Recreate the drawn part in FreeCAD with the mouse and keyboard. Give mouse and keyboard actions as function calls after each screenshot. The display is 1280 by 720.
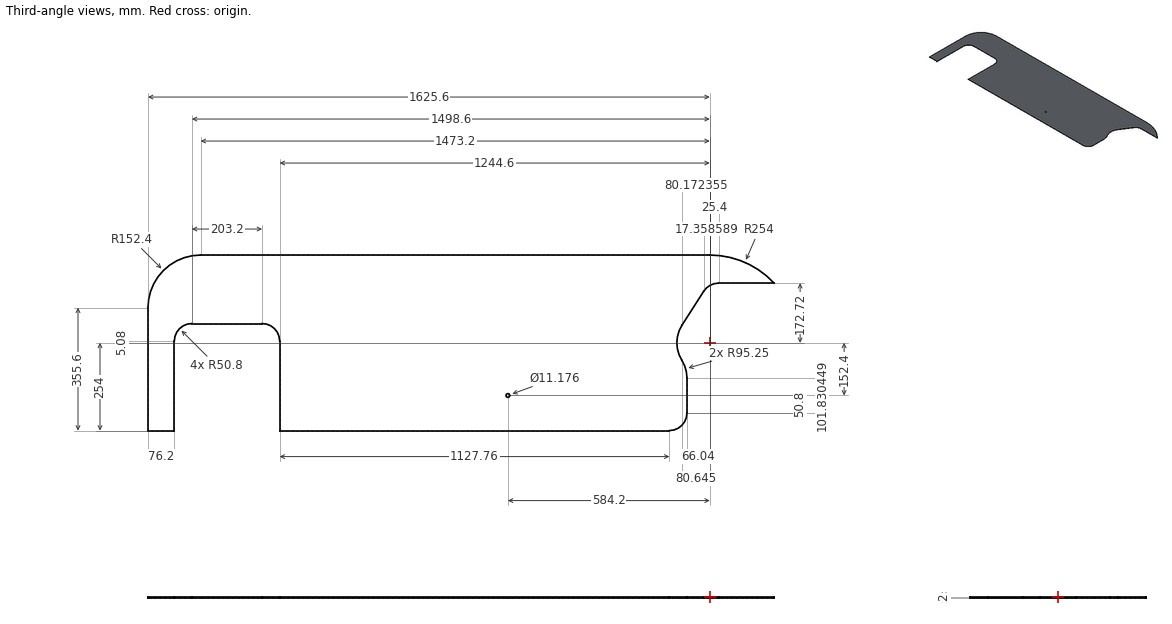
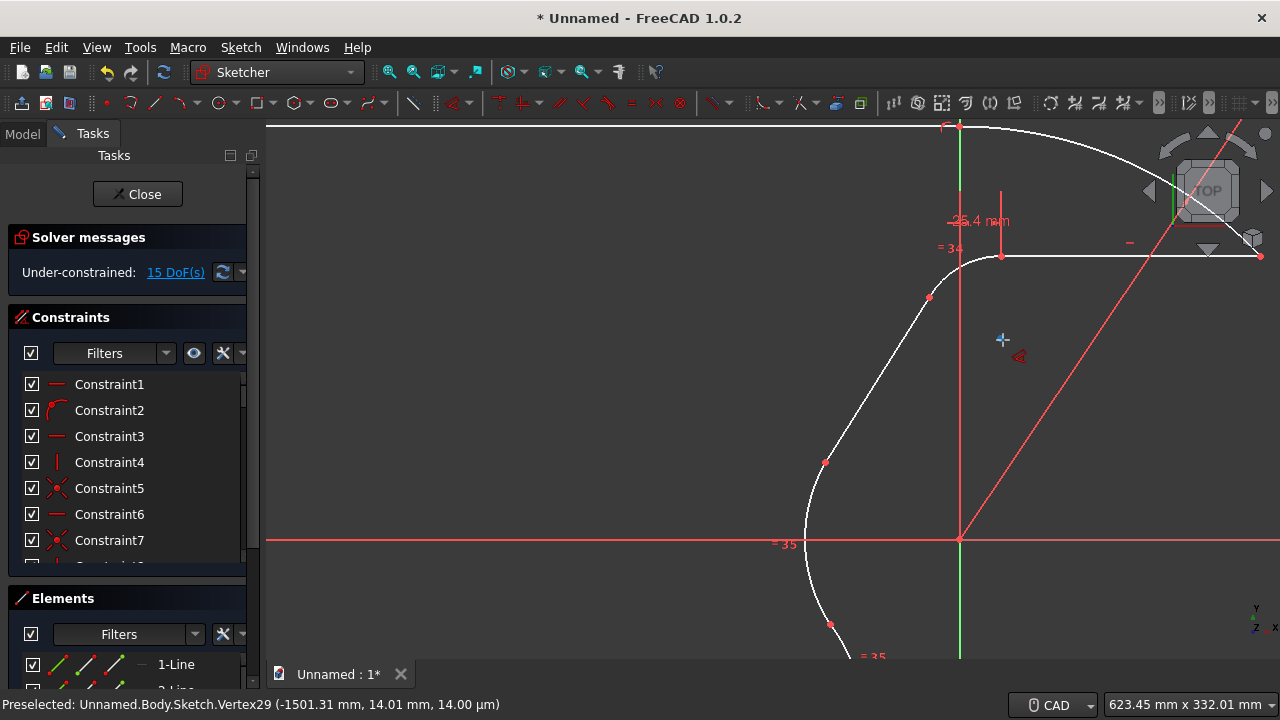
click(1001, 339)
click(980, 305)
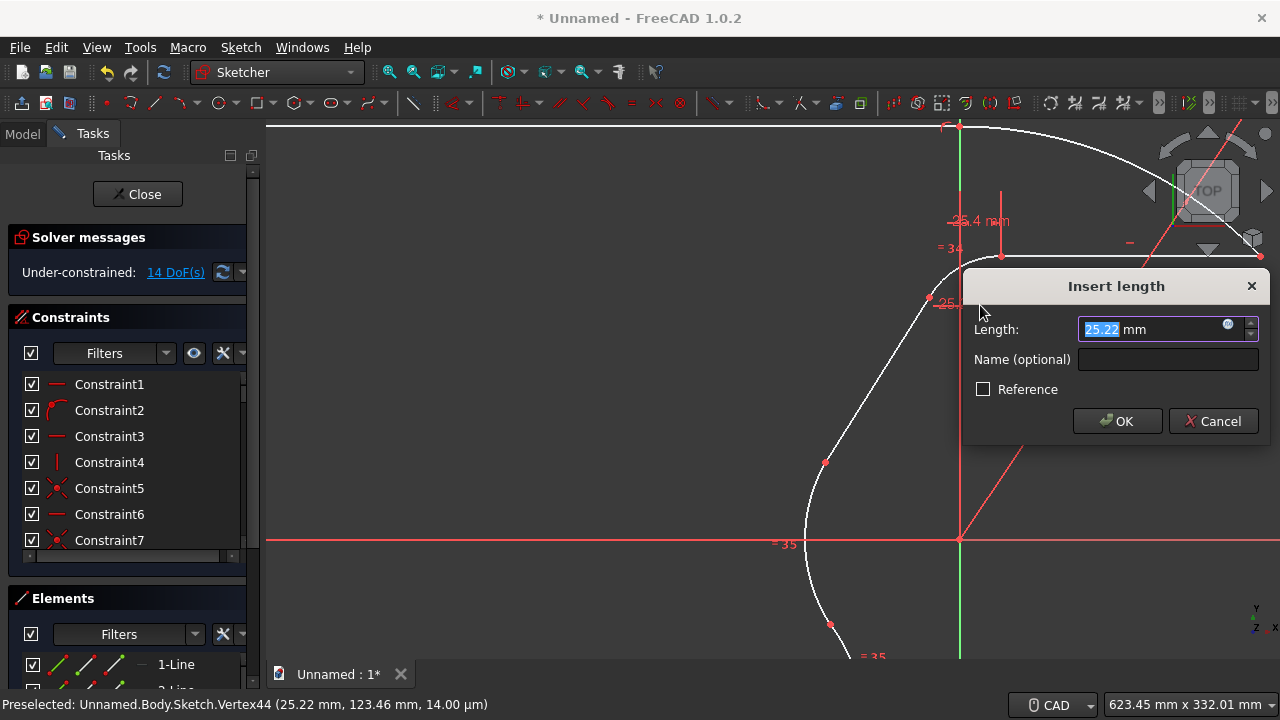
text(25.4)
key(Return)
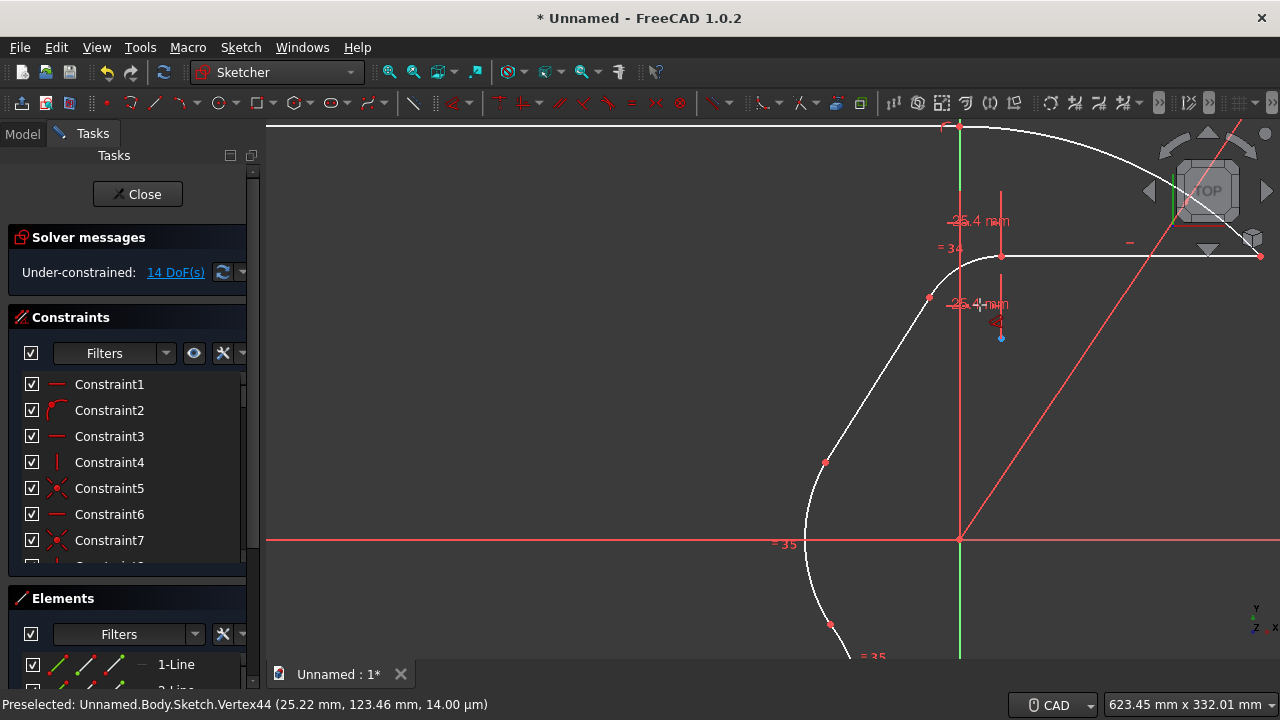
scroll(936, 351, down, 8)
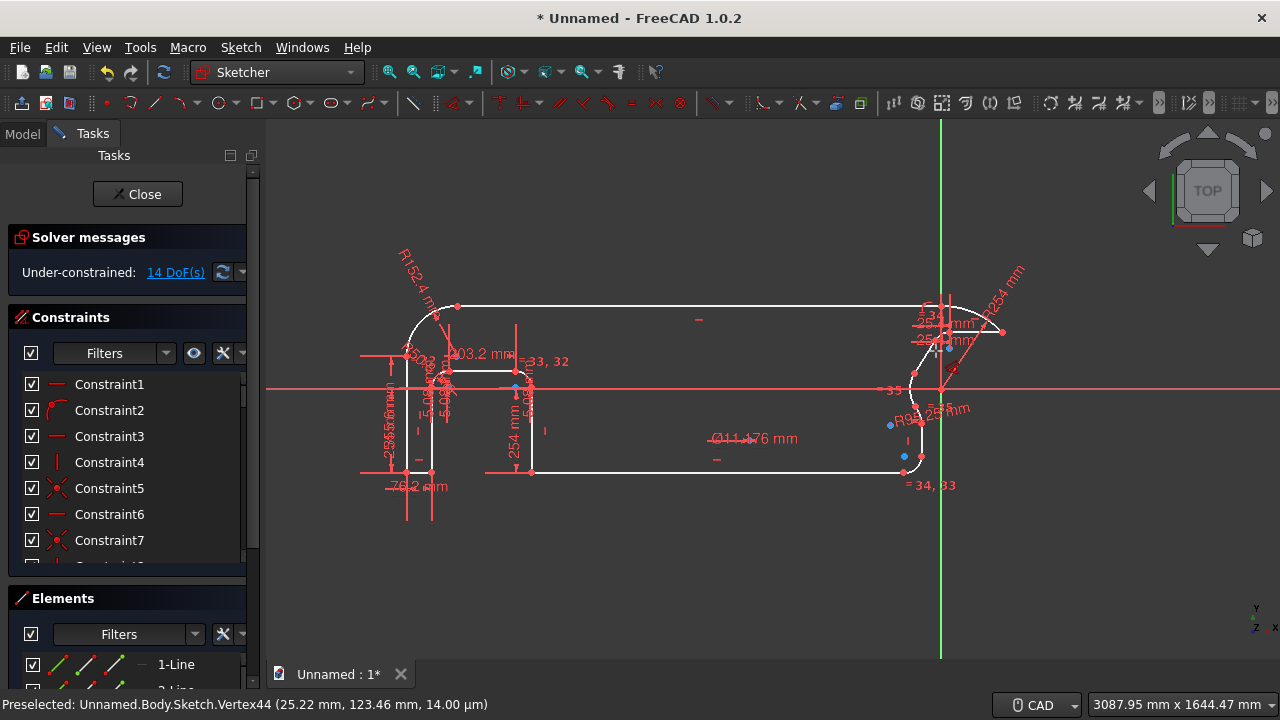
click(750, 441)
click(846, 355)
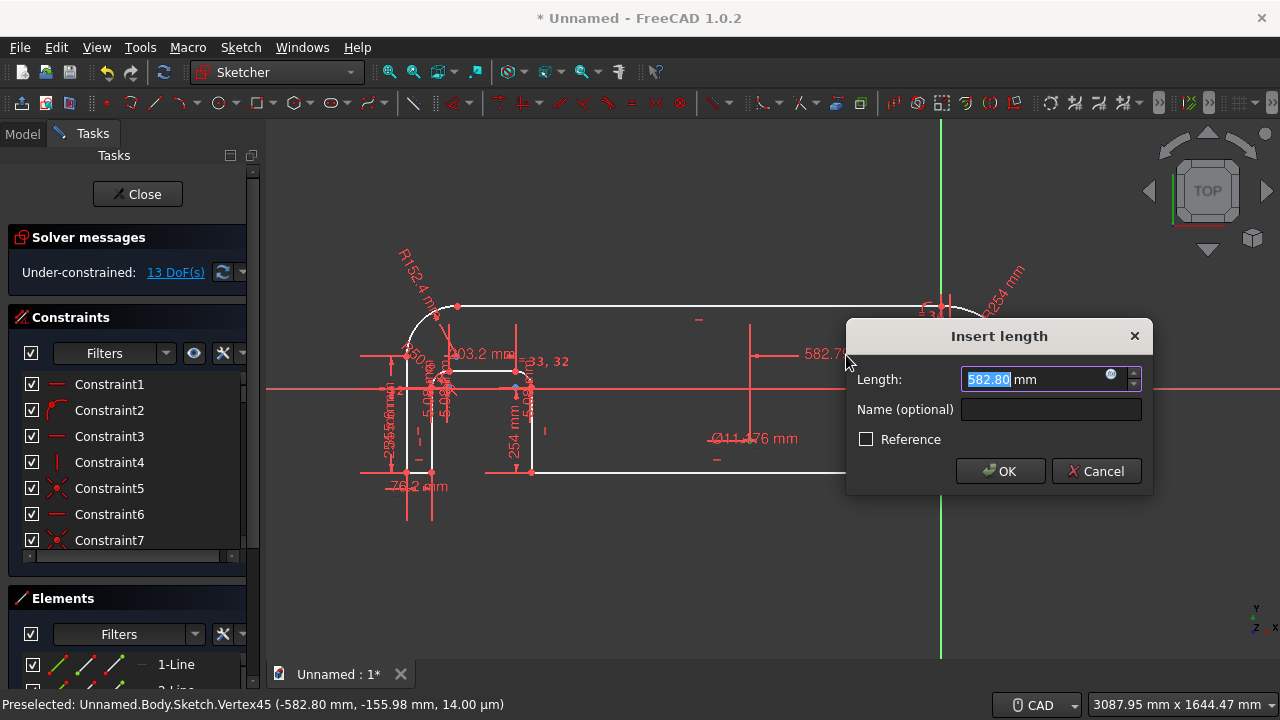
text(584.2)
key(Return)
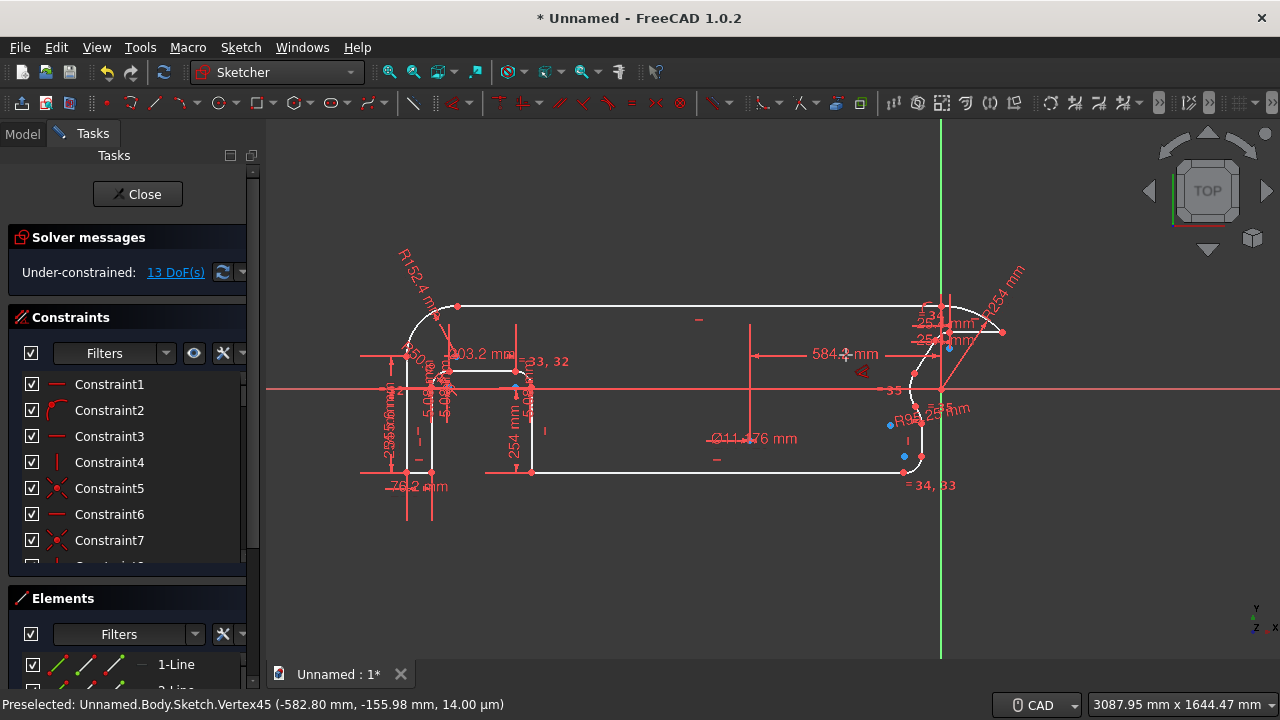
click(750, 441)
click(716, 415)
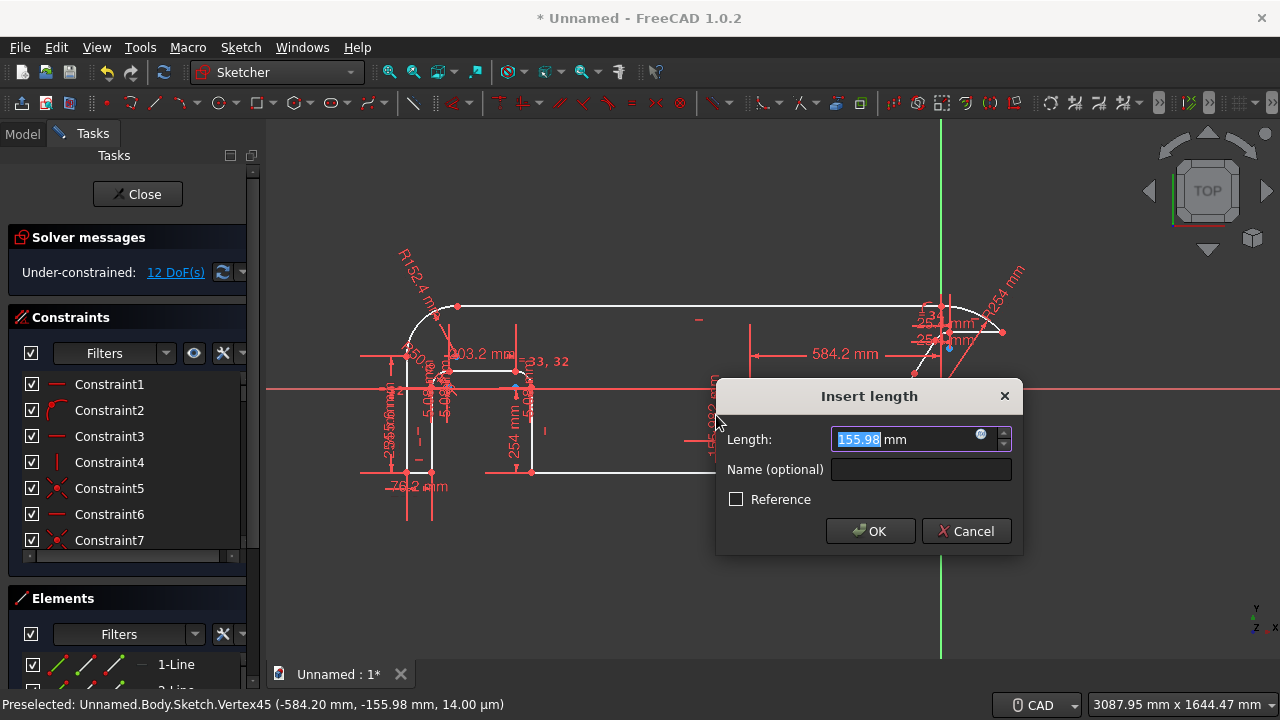
text(152.4)
key(Return)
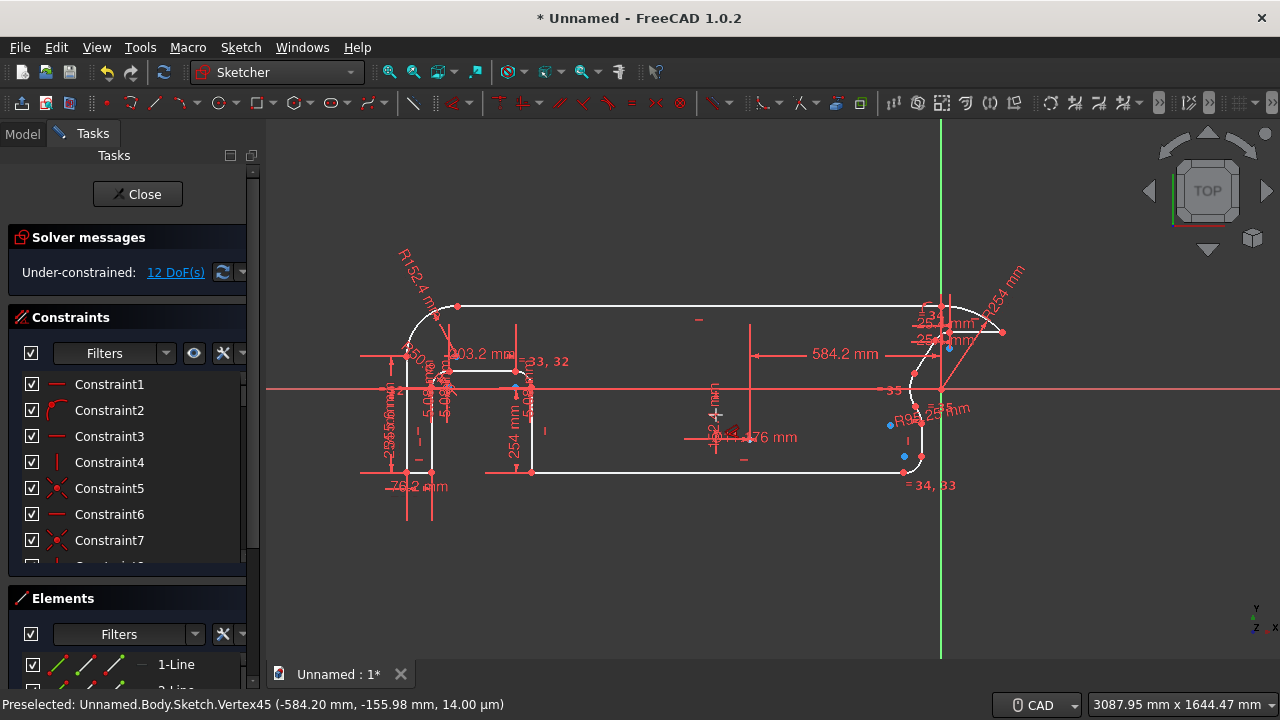
scroll(922, 457, up, 5)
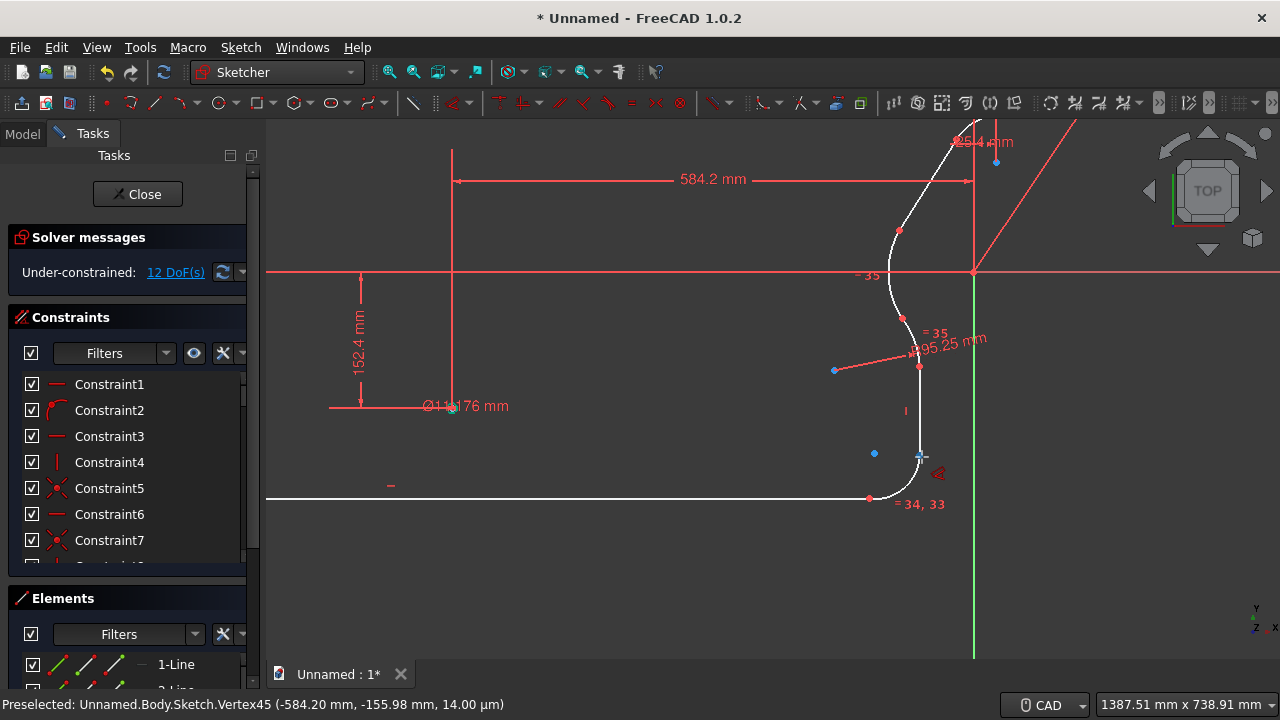
click(920, 456)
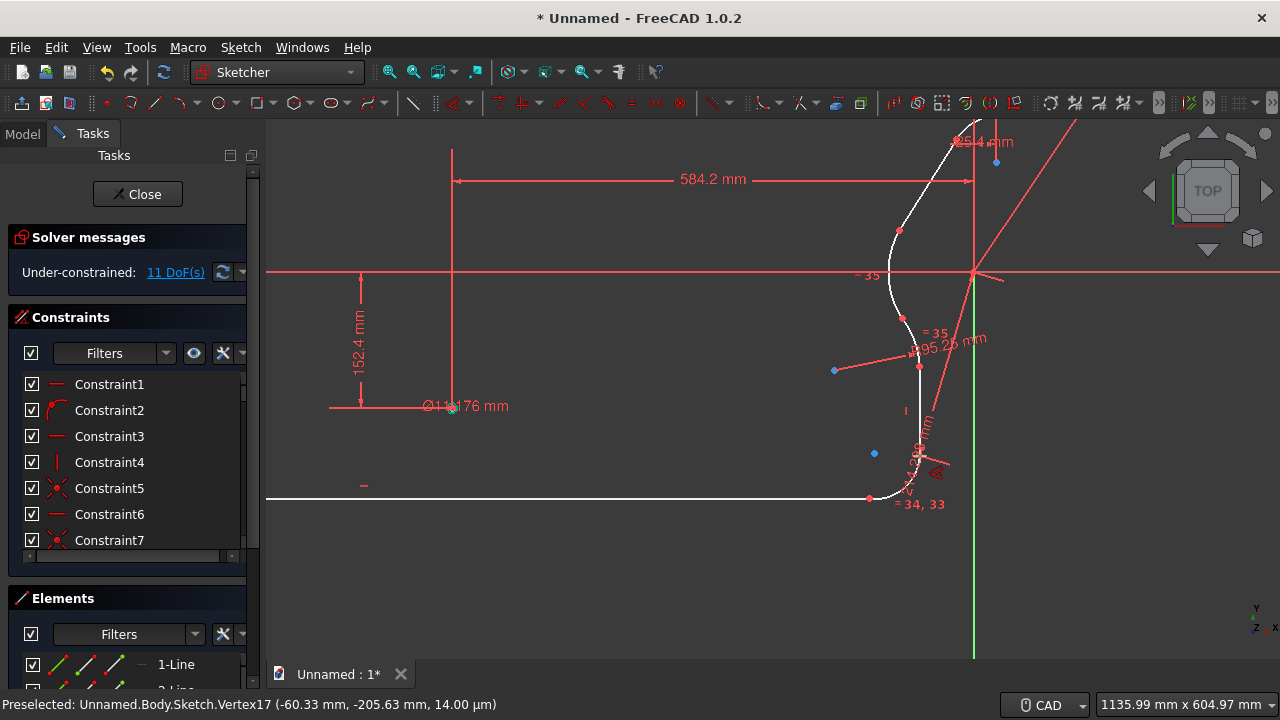
click(452, 408)
click(954, 432)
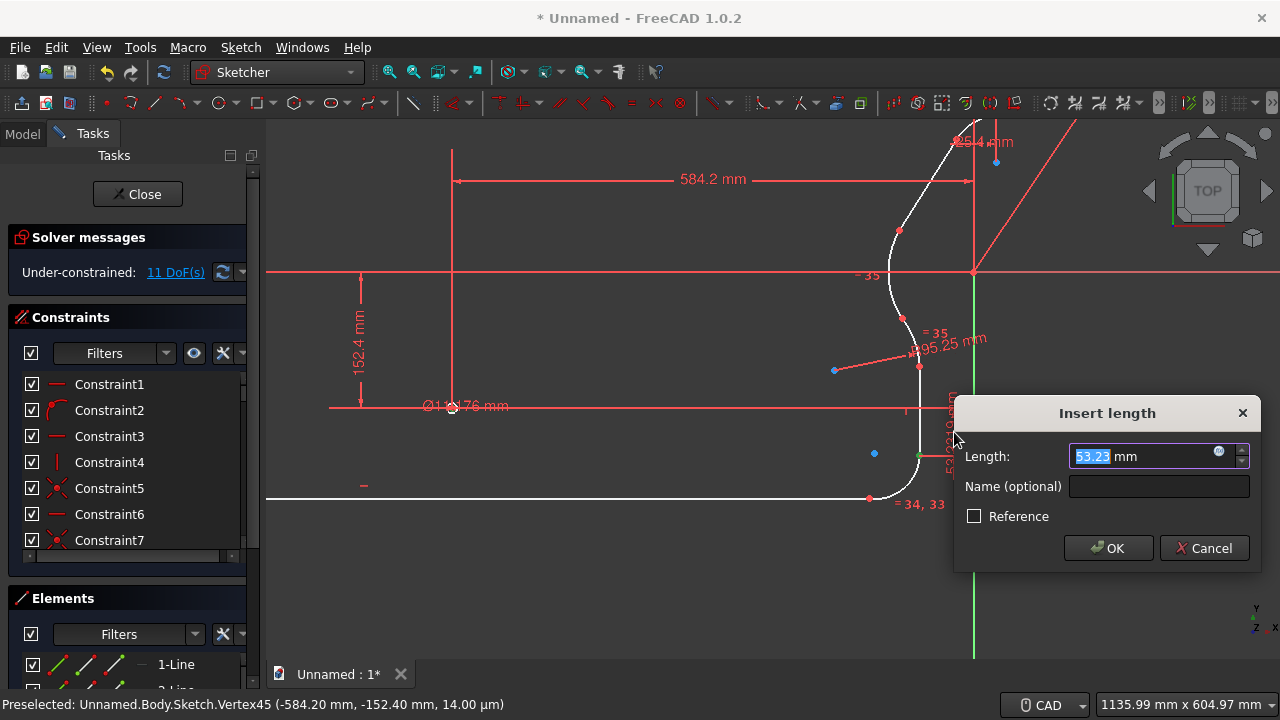
text(50.8)
key(Return)